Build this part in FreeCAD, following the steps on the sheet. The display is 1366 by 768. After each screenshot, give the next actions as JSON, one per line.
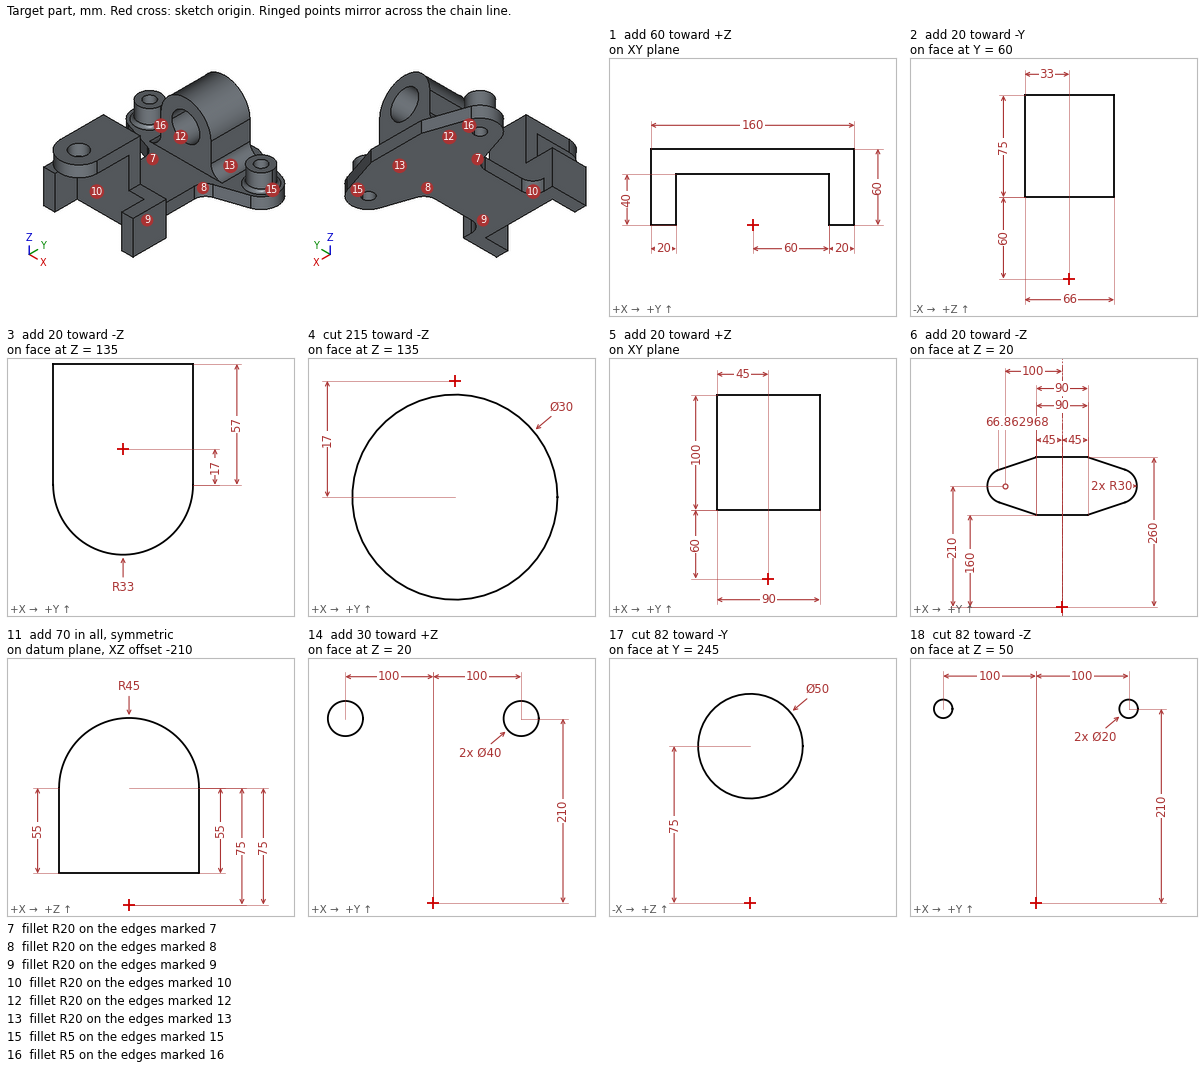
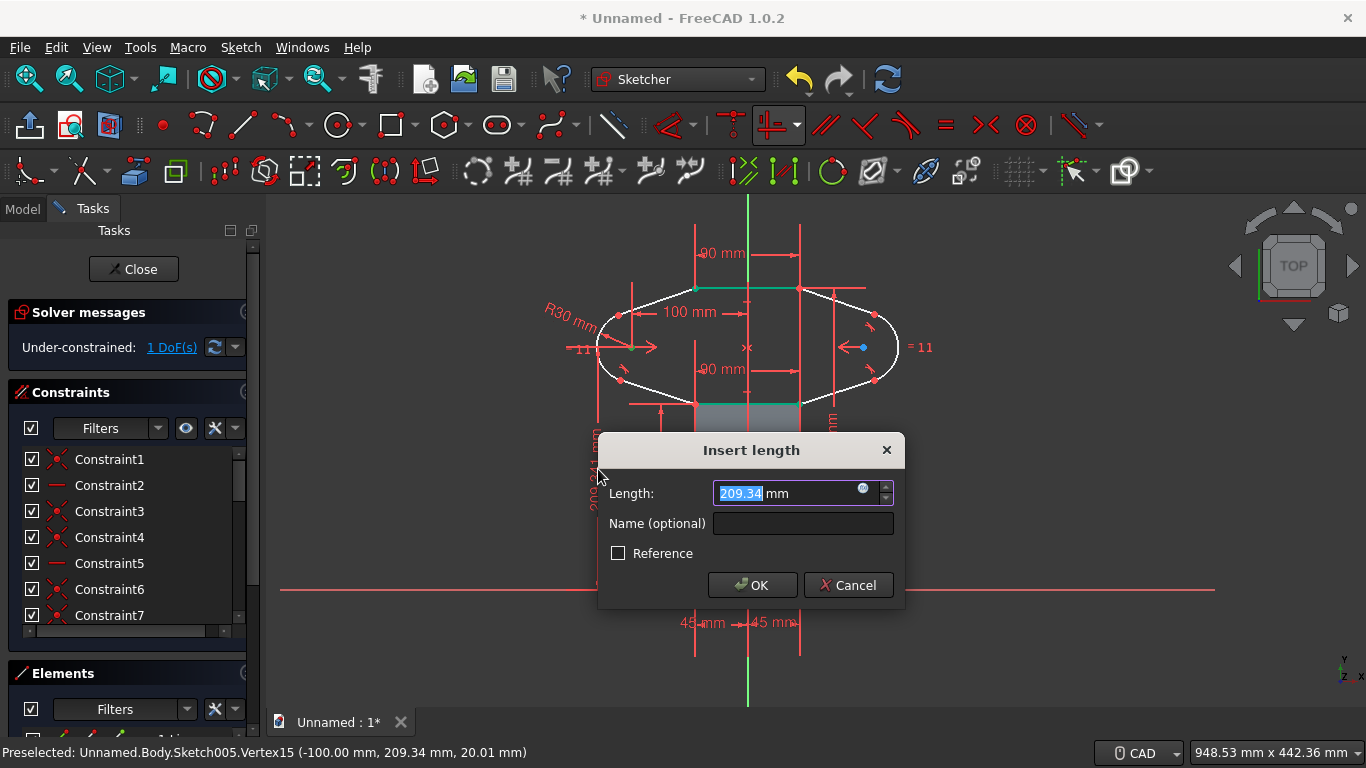
{"action": "type", "text": "210"}
{"action": "key", "text": "Return"}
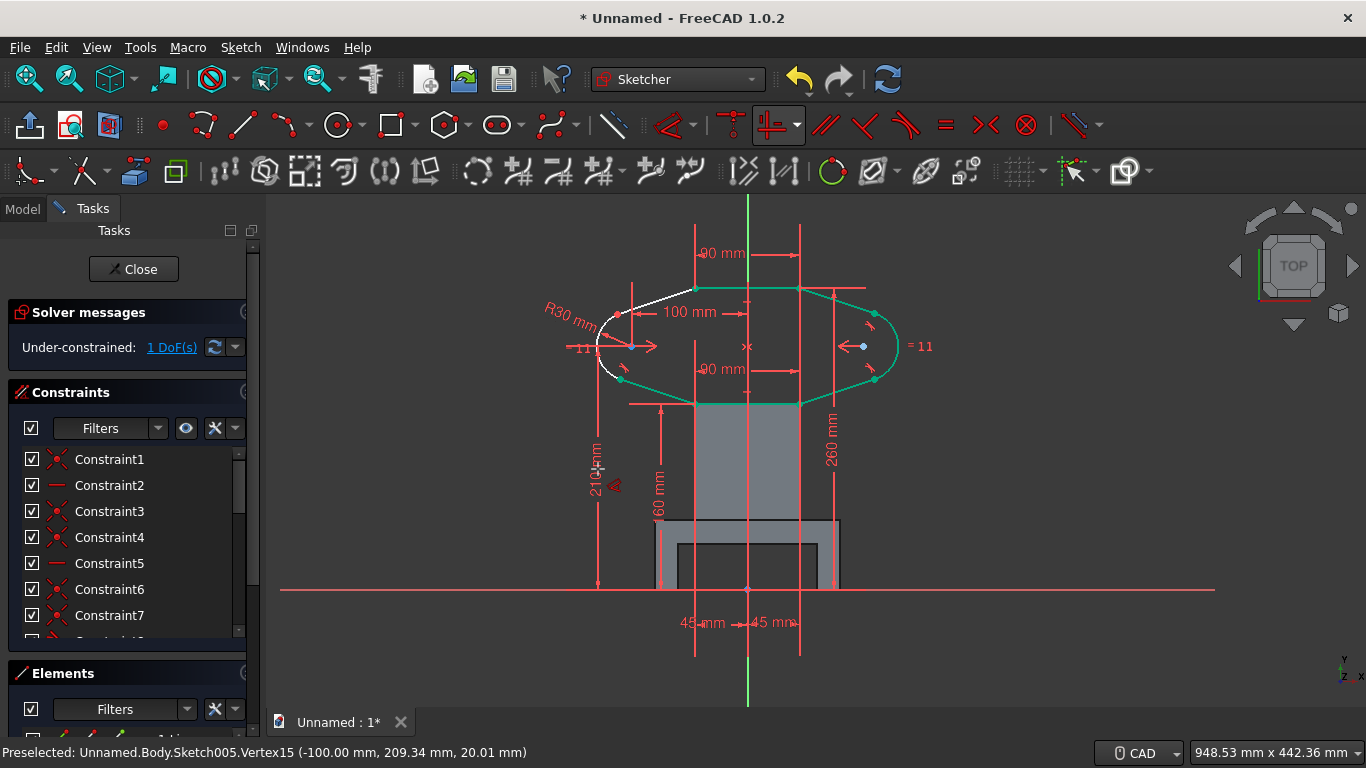
{"action": "left_click", "coordinate": [672, 296]}
{"action": "left_click", "coordinate": [639, 254]}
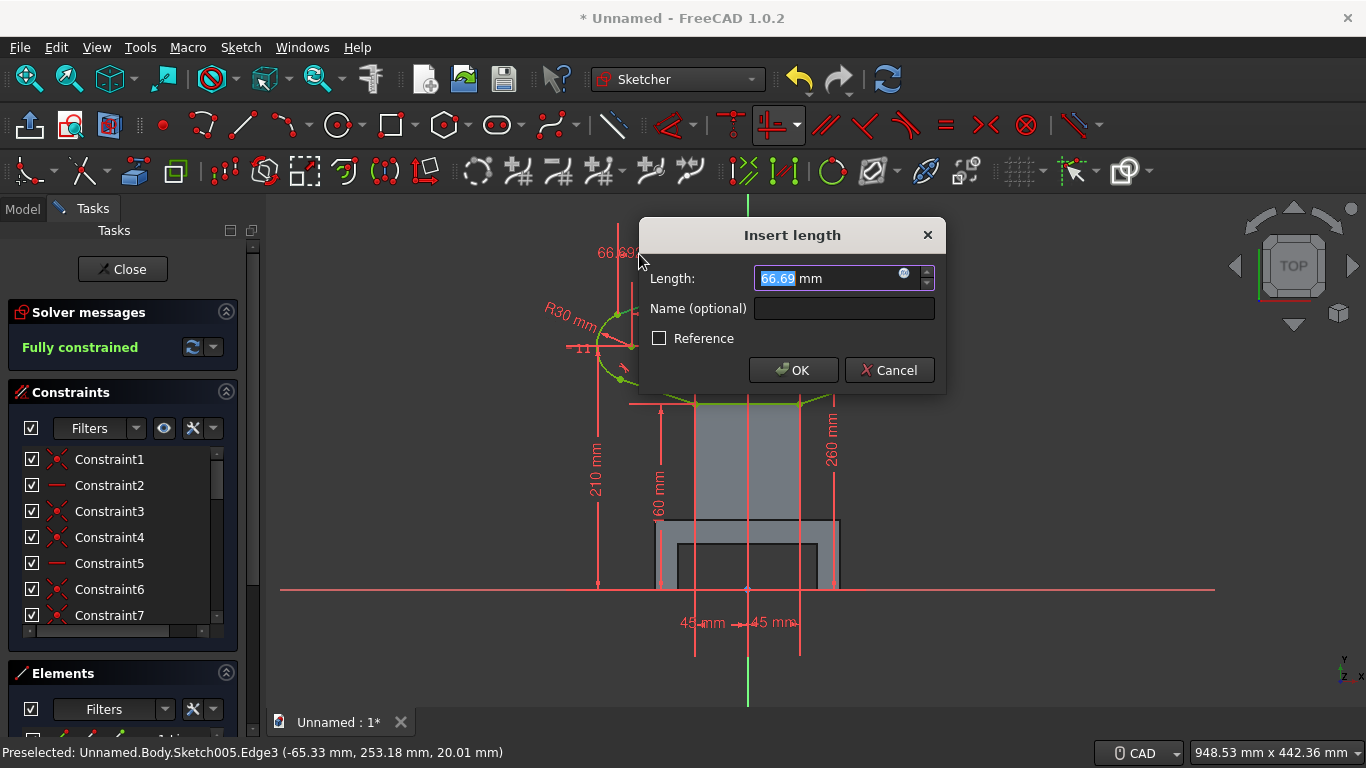
{"action": "type", "text": "66.862968"}
{"action": "key", "text": "Return"}
{"action": "key", "text": "Escape"}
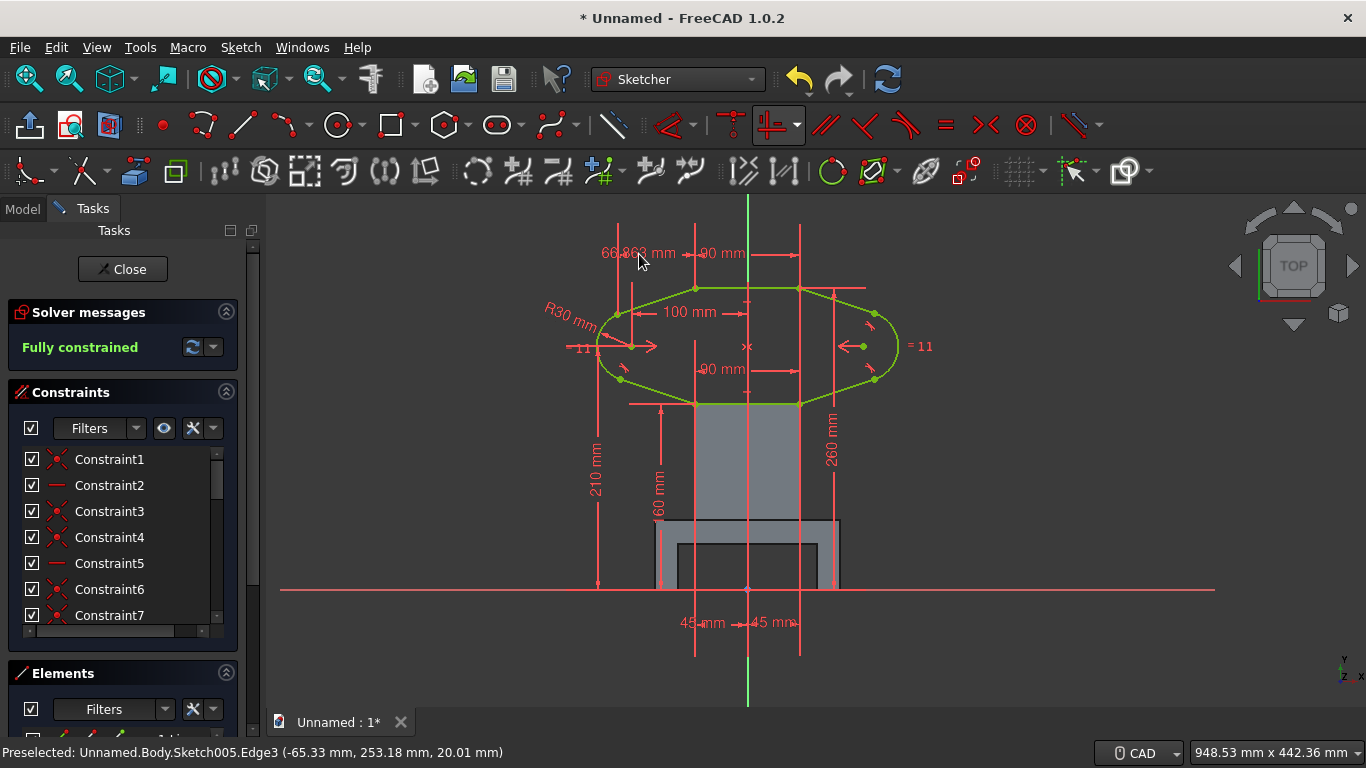
{"action": "left_click", "coordinate": [123, 269]}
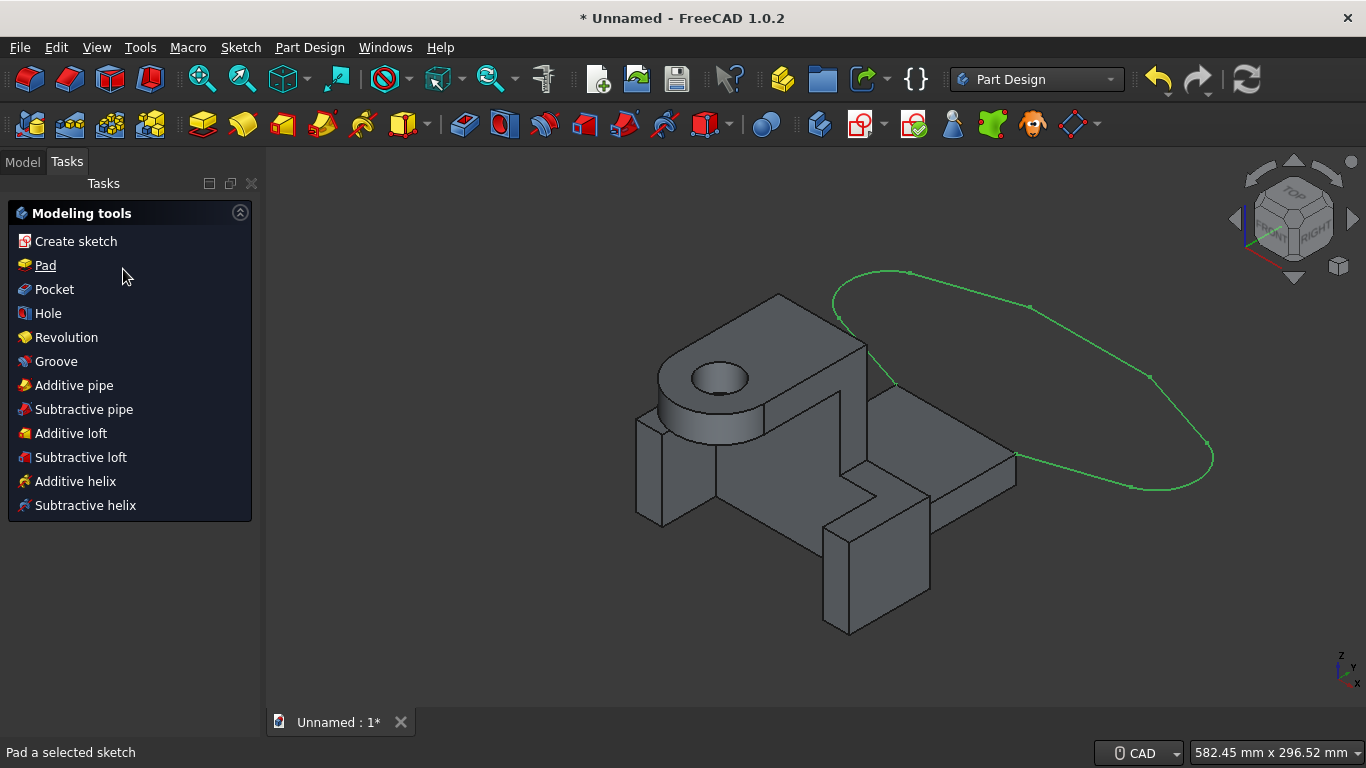
{"action": "left_click", "coordinate": [204, 124]}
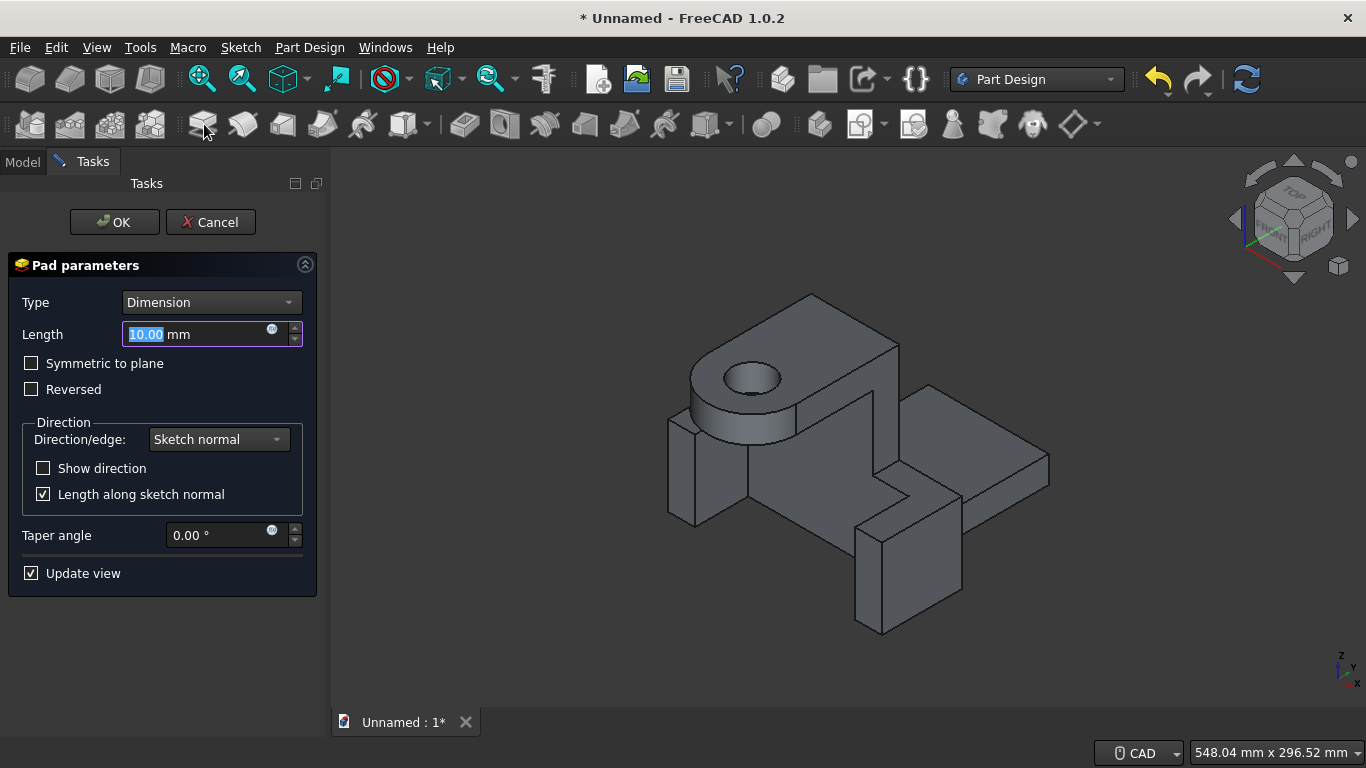
{"action": "type", "text": "20"}
{"action": "key", "text": "Tab"}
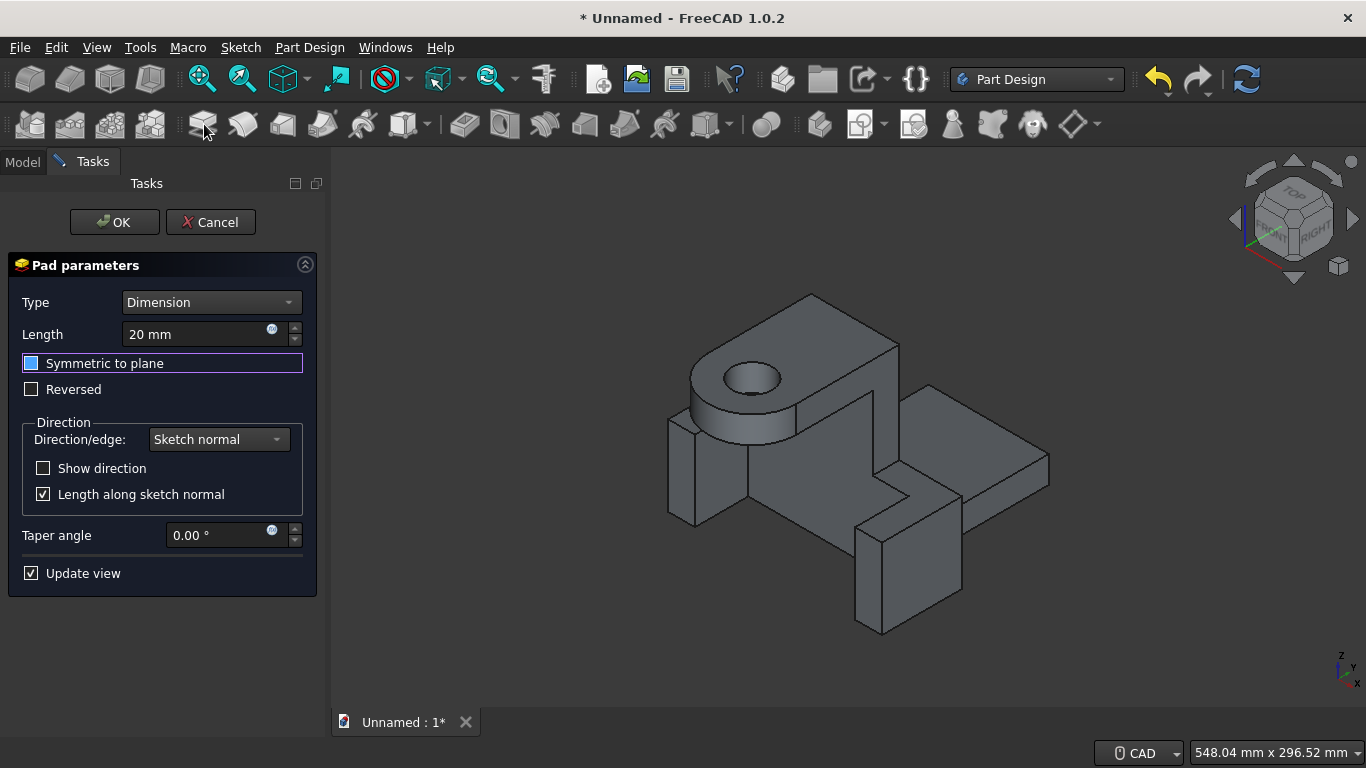
{"action": "left_click", "coordinate": [30, 389]}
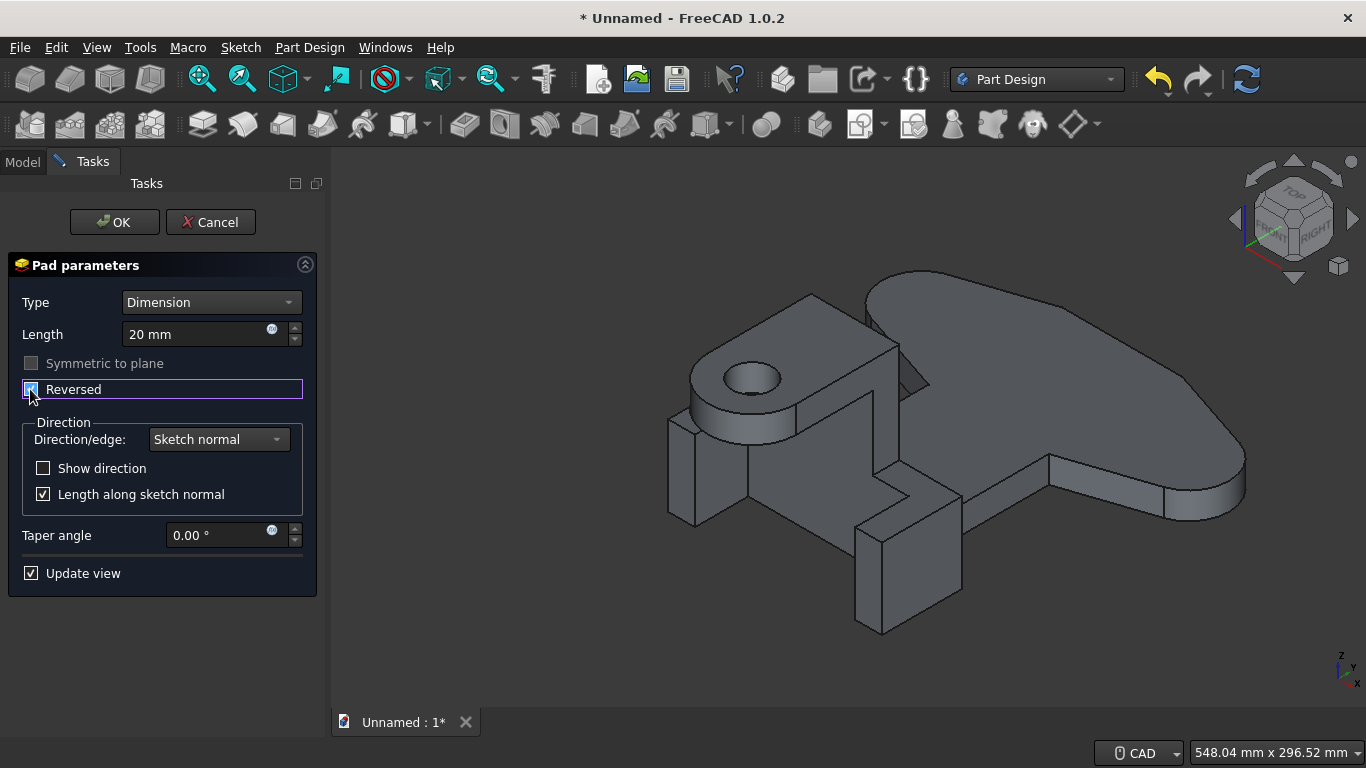
{"action": "left_click", "coordinate": [115, 222]}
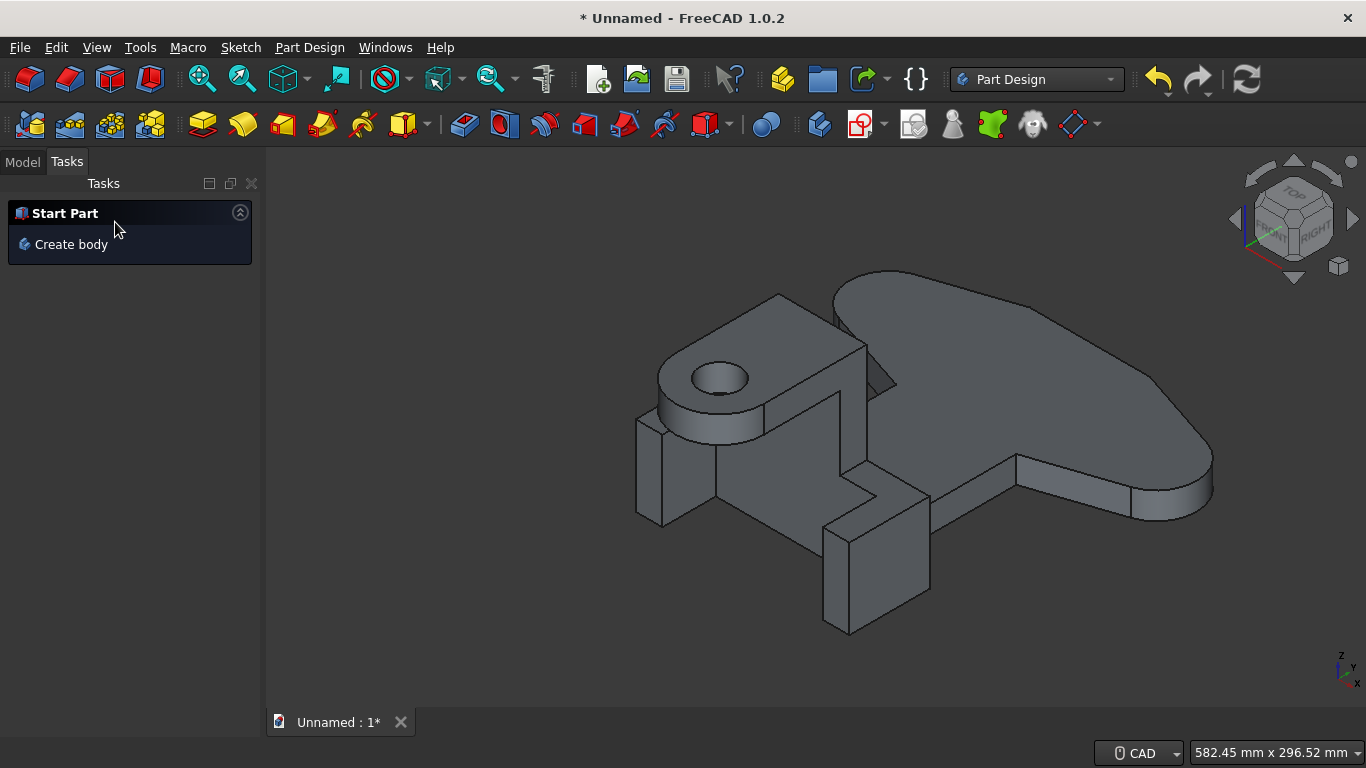
{"action": "key", "text": "v f"}